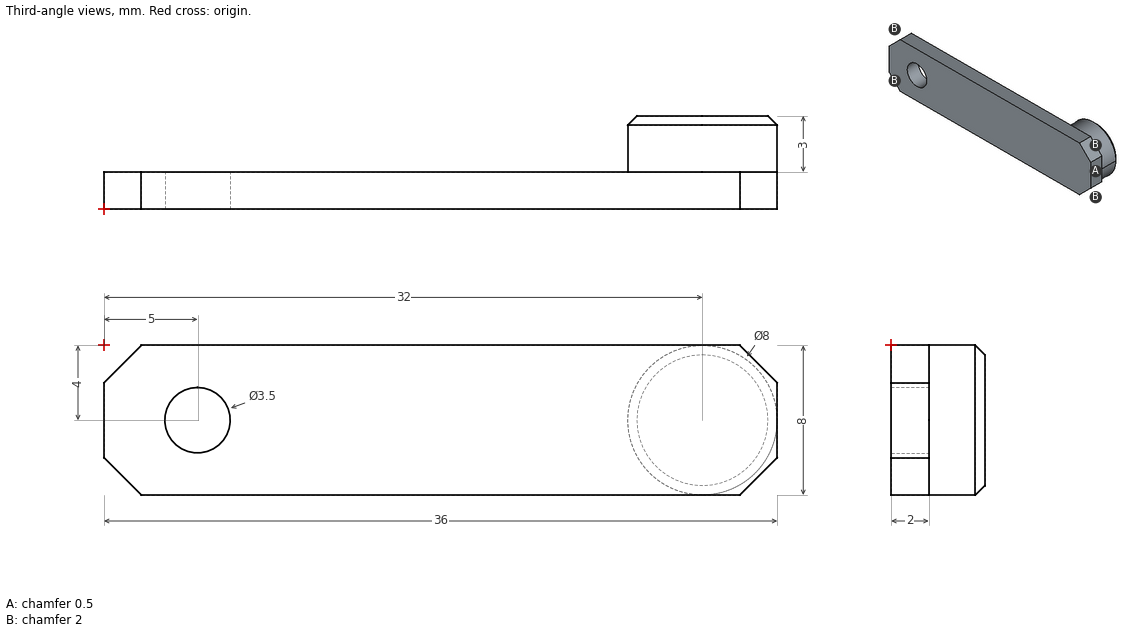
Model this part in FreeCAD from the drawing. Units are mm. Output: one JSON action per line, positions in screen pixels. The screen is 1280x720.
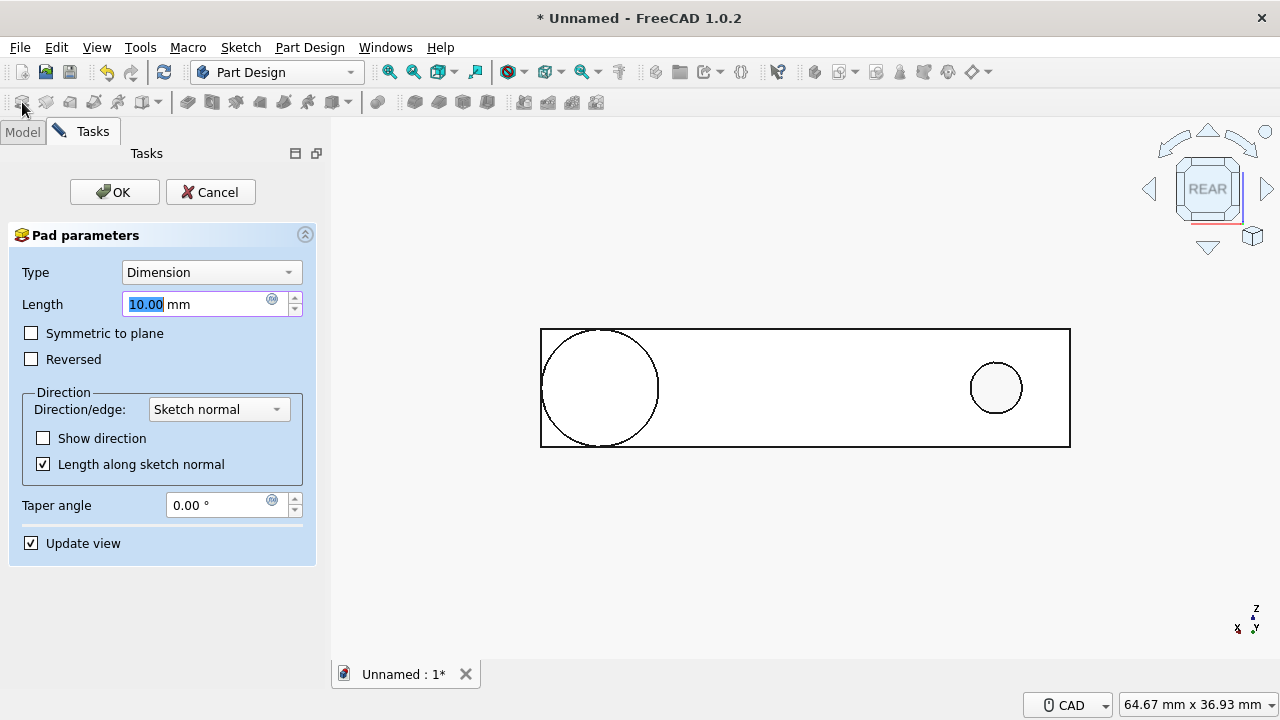
{"action": "type", "text": "3"}
{"action": "key", "text": "Tab"}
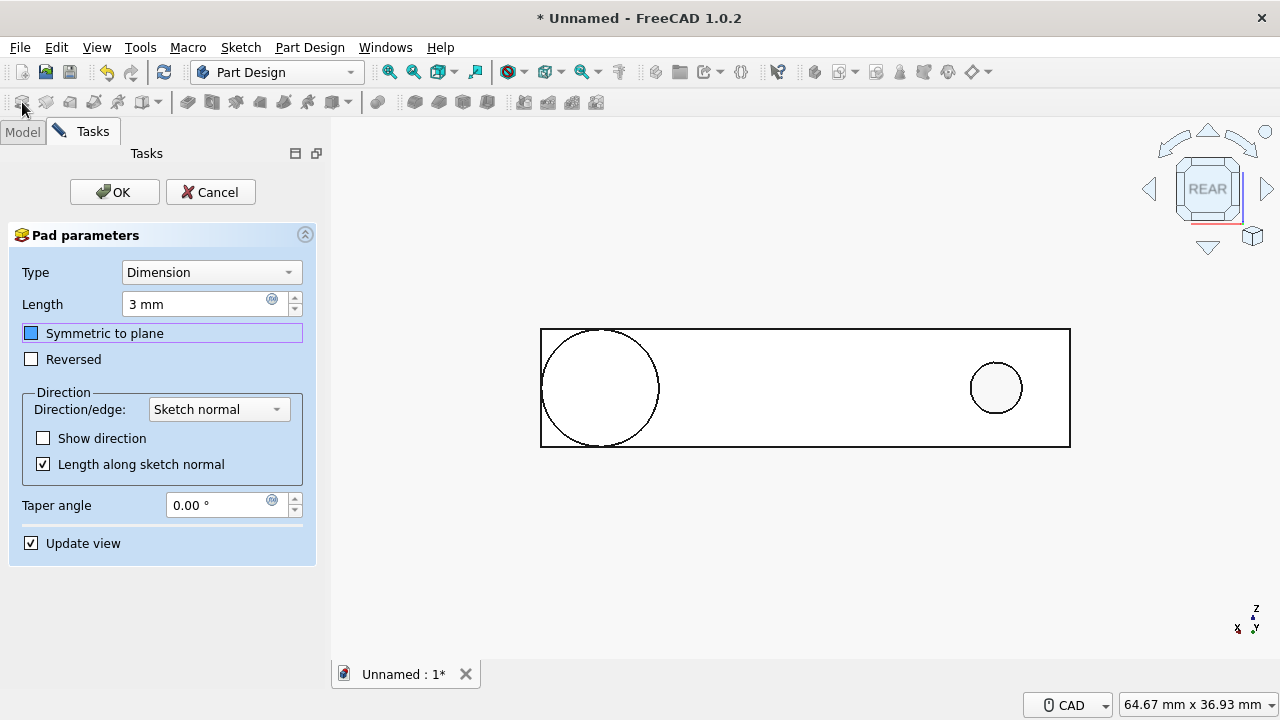
{"action": "left_click", "coordinate": [115, 192]}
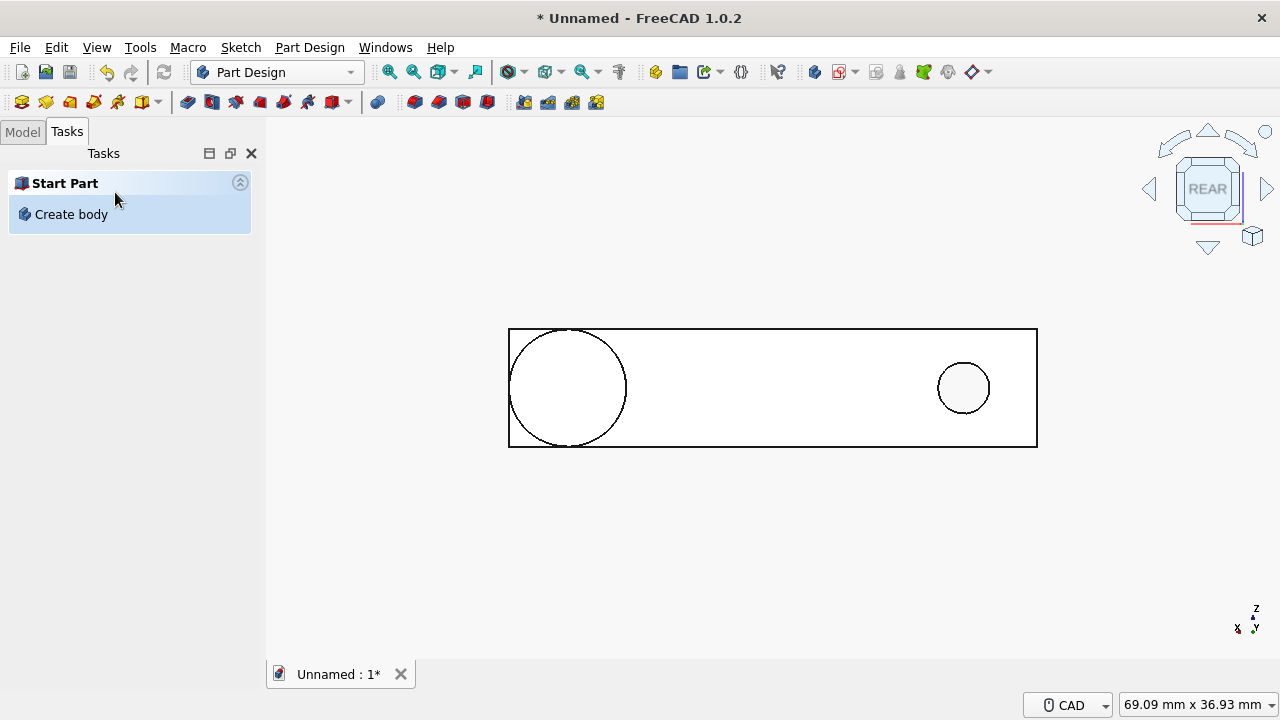
{"action": "left_click", "coordinate": [626, 387]}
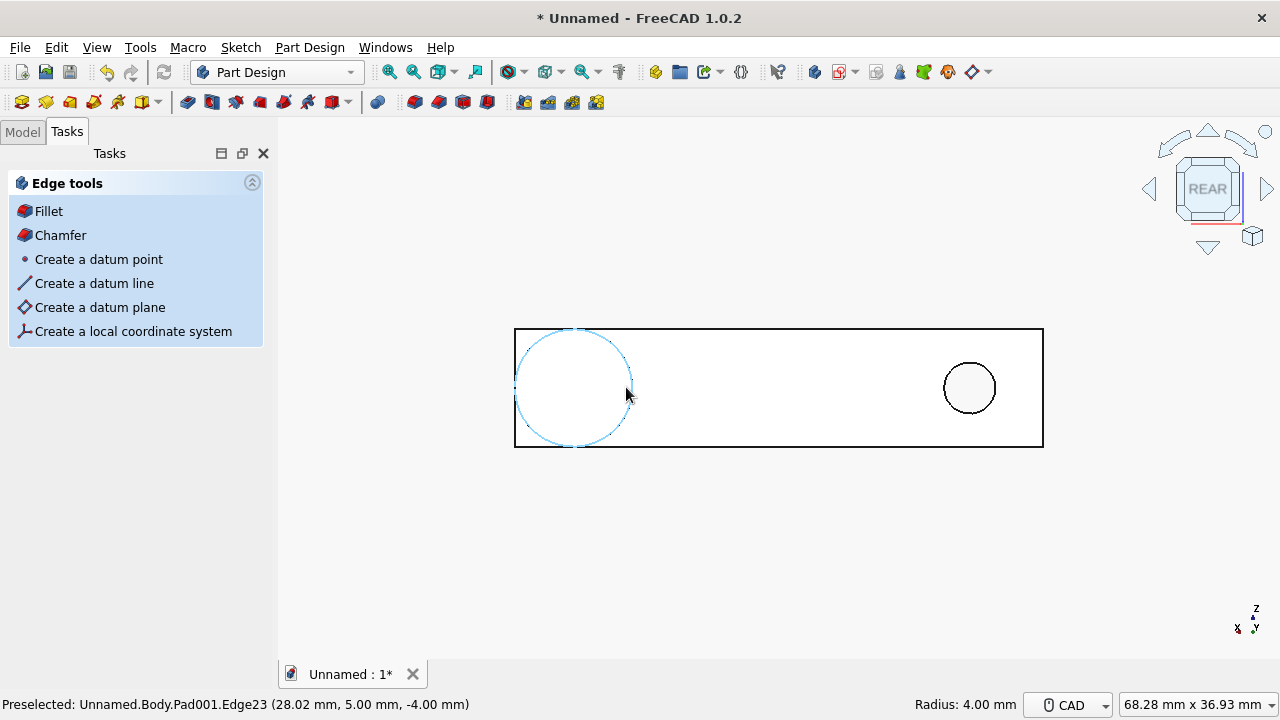
{"action": "left_click", "coordinate": [440, 102]}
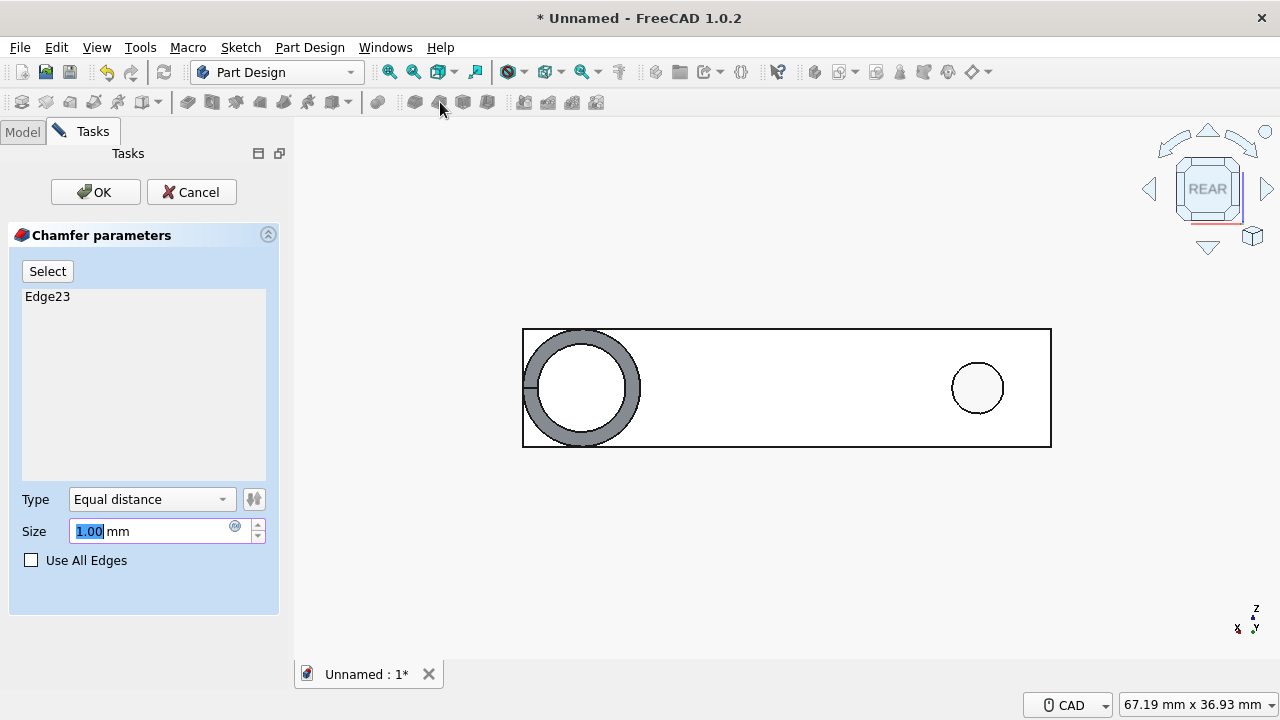
{"action": "type", "text": "0.5"}
{"action": "key", "text": "Tab"}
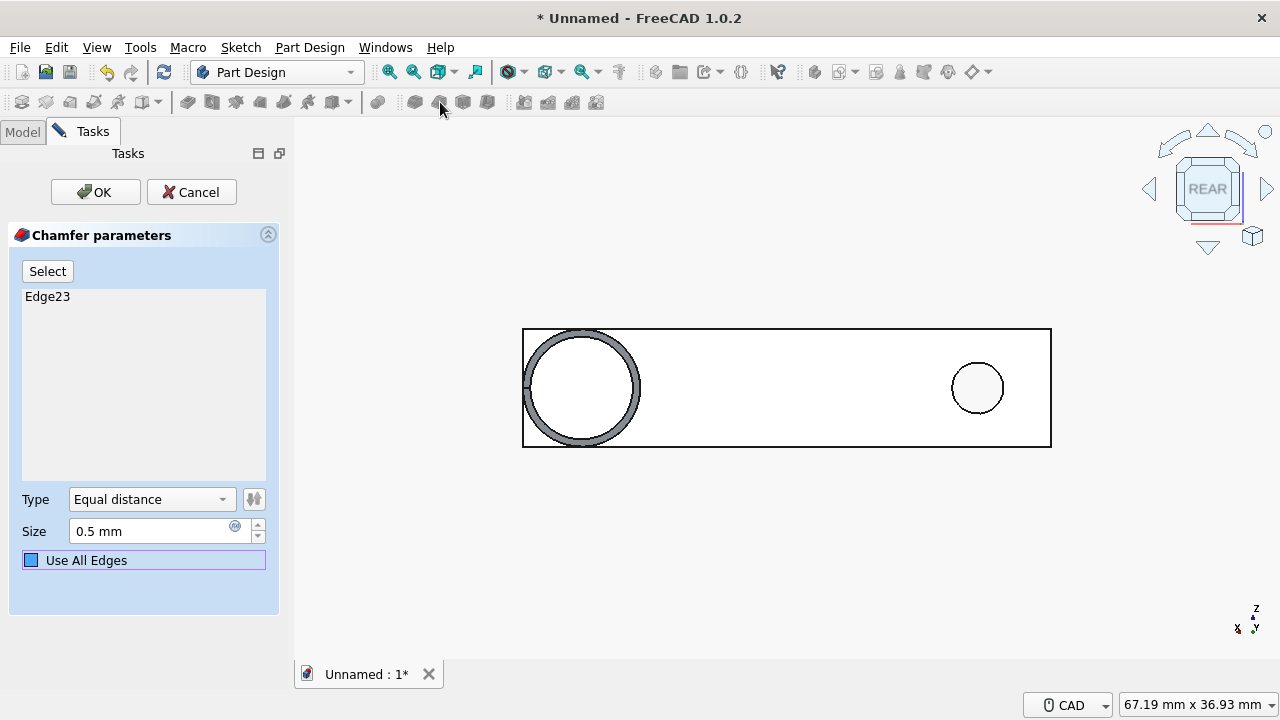
{"action": "left_click", "coordinate": [96, 192]}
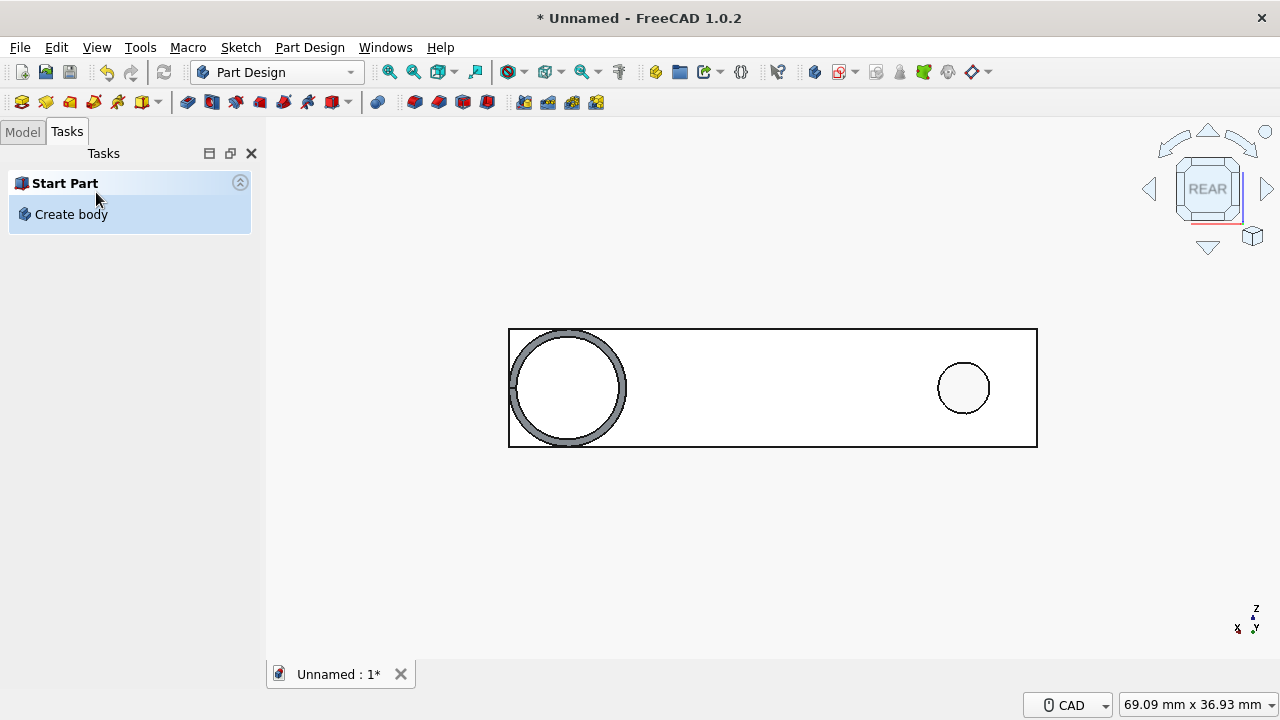
{"action": "key", "text": "0"}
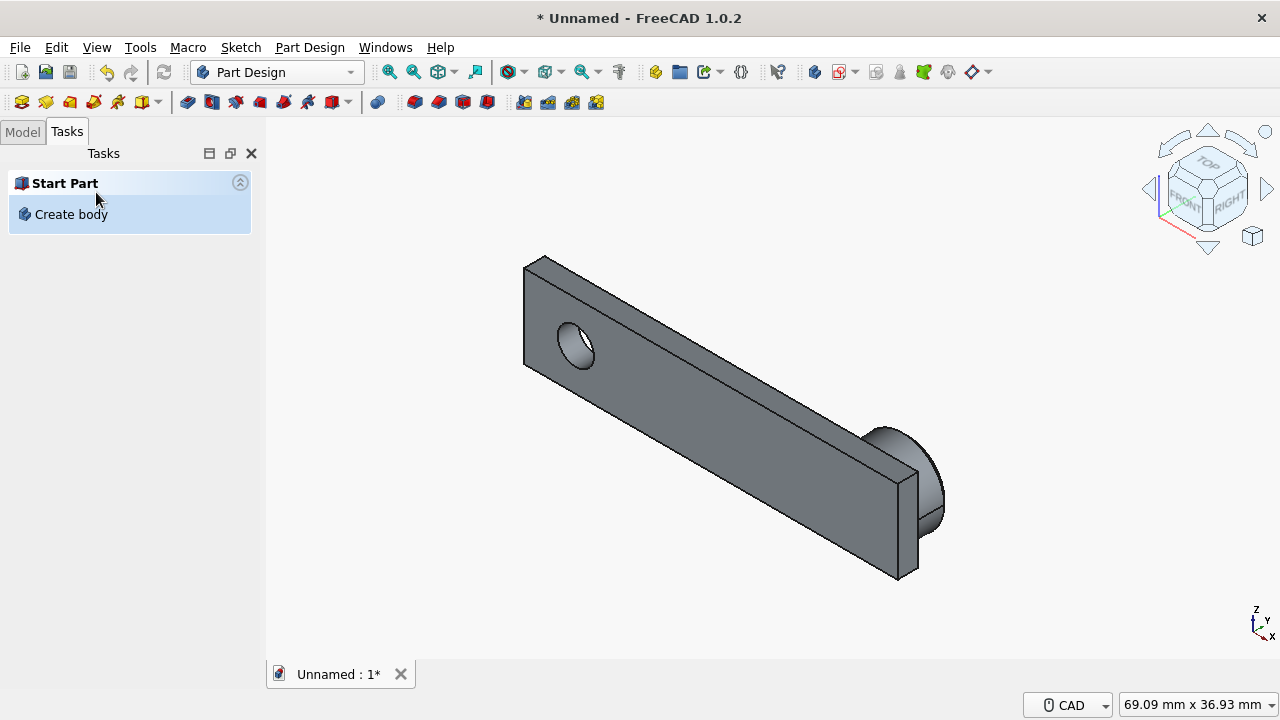
{"action": "left_click", "coordinate": [908, 477]}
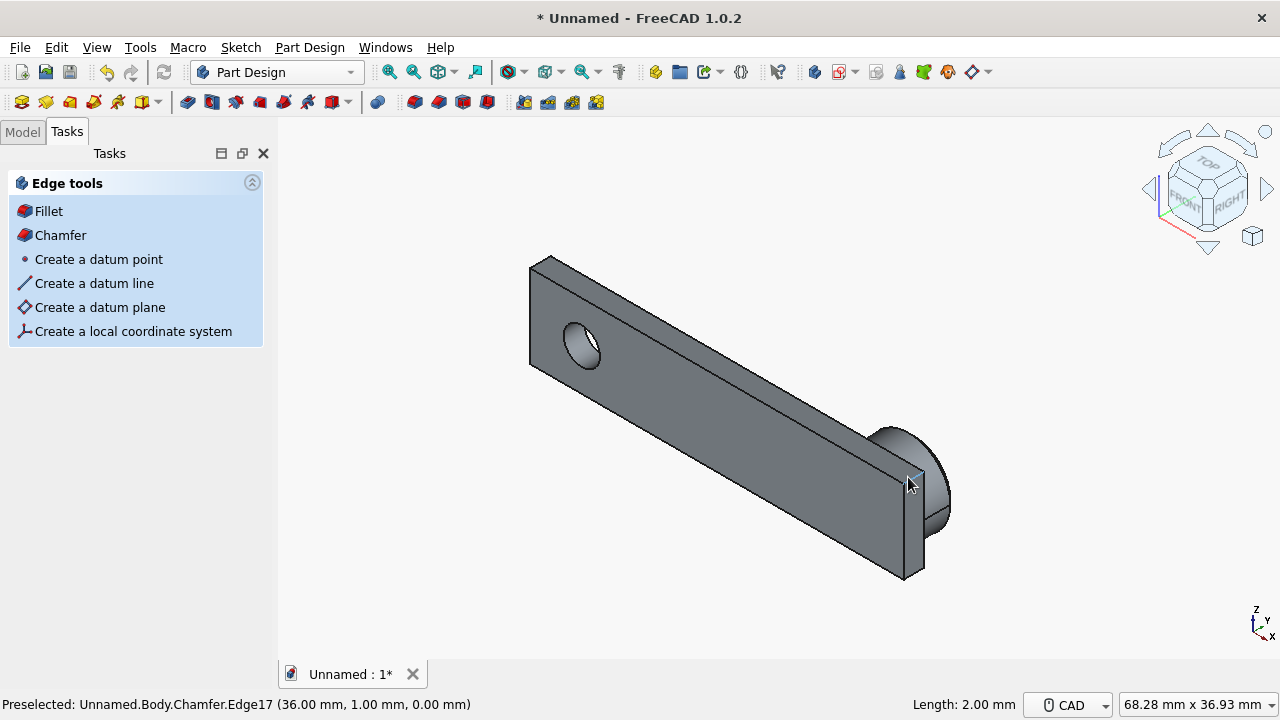
{"action": "key", "text": "2"}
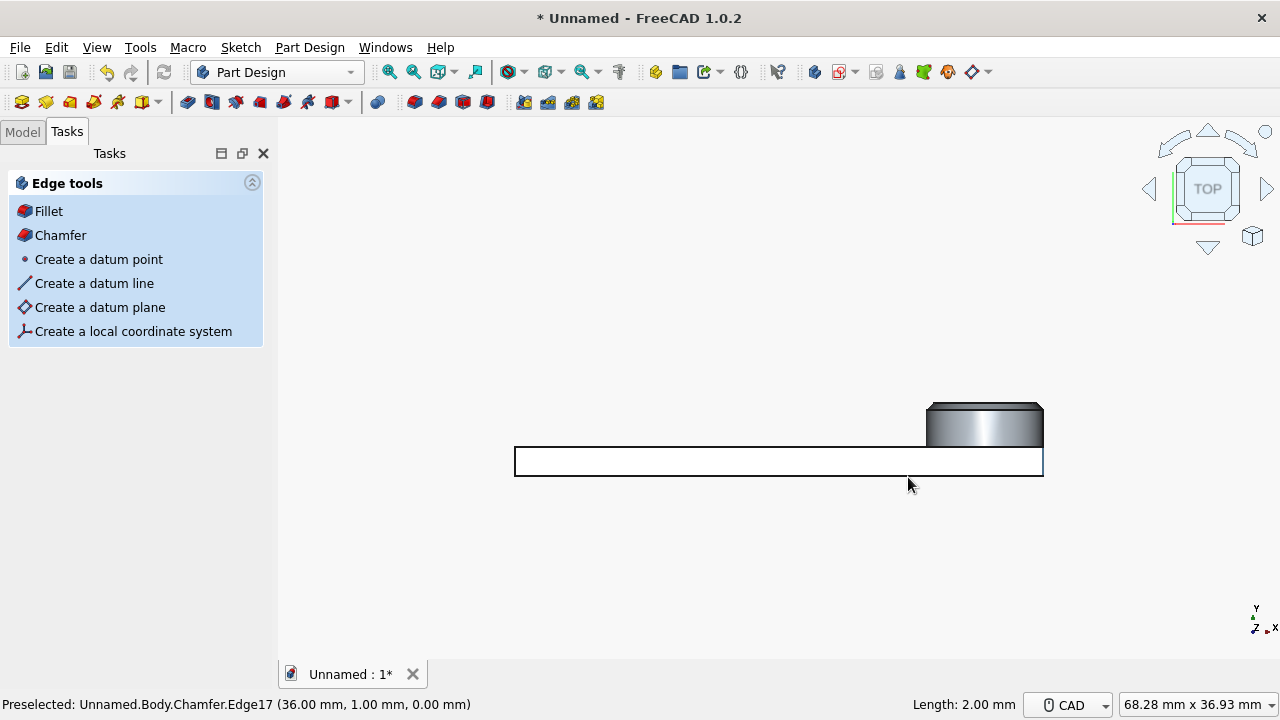
{"action": "left_click", "coordinate": [515, 457], "text": "ctrl"}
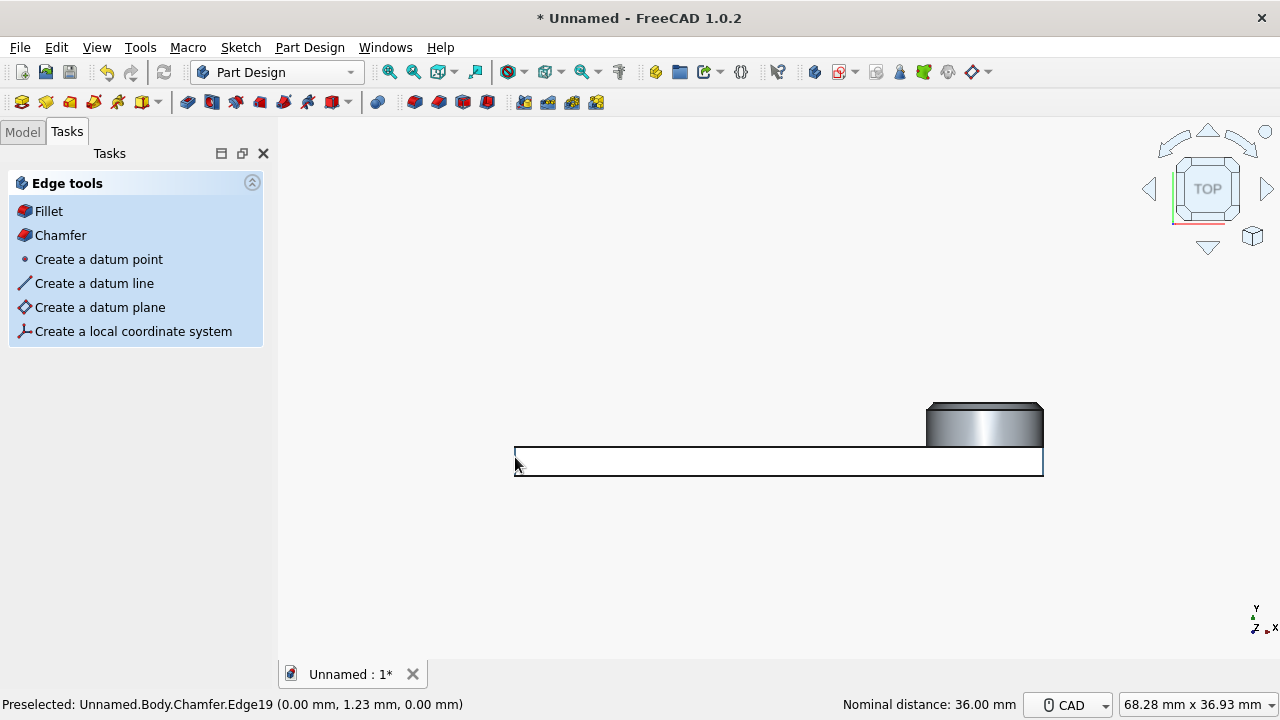
{"action": "key", "text": "1"}